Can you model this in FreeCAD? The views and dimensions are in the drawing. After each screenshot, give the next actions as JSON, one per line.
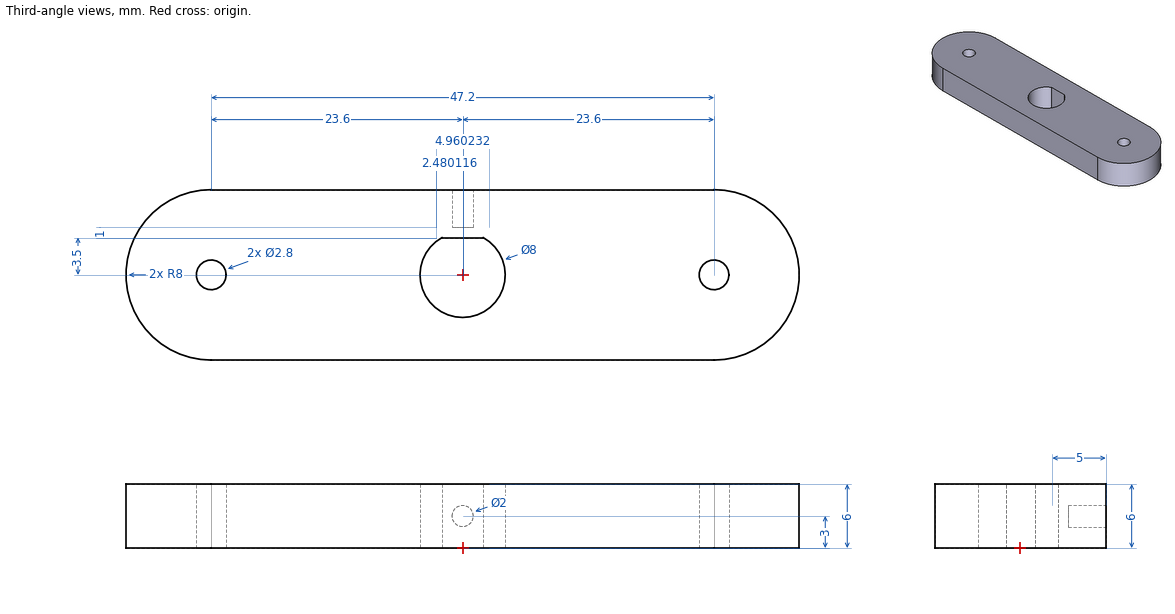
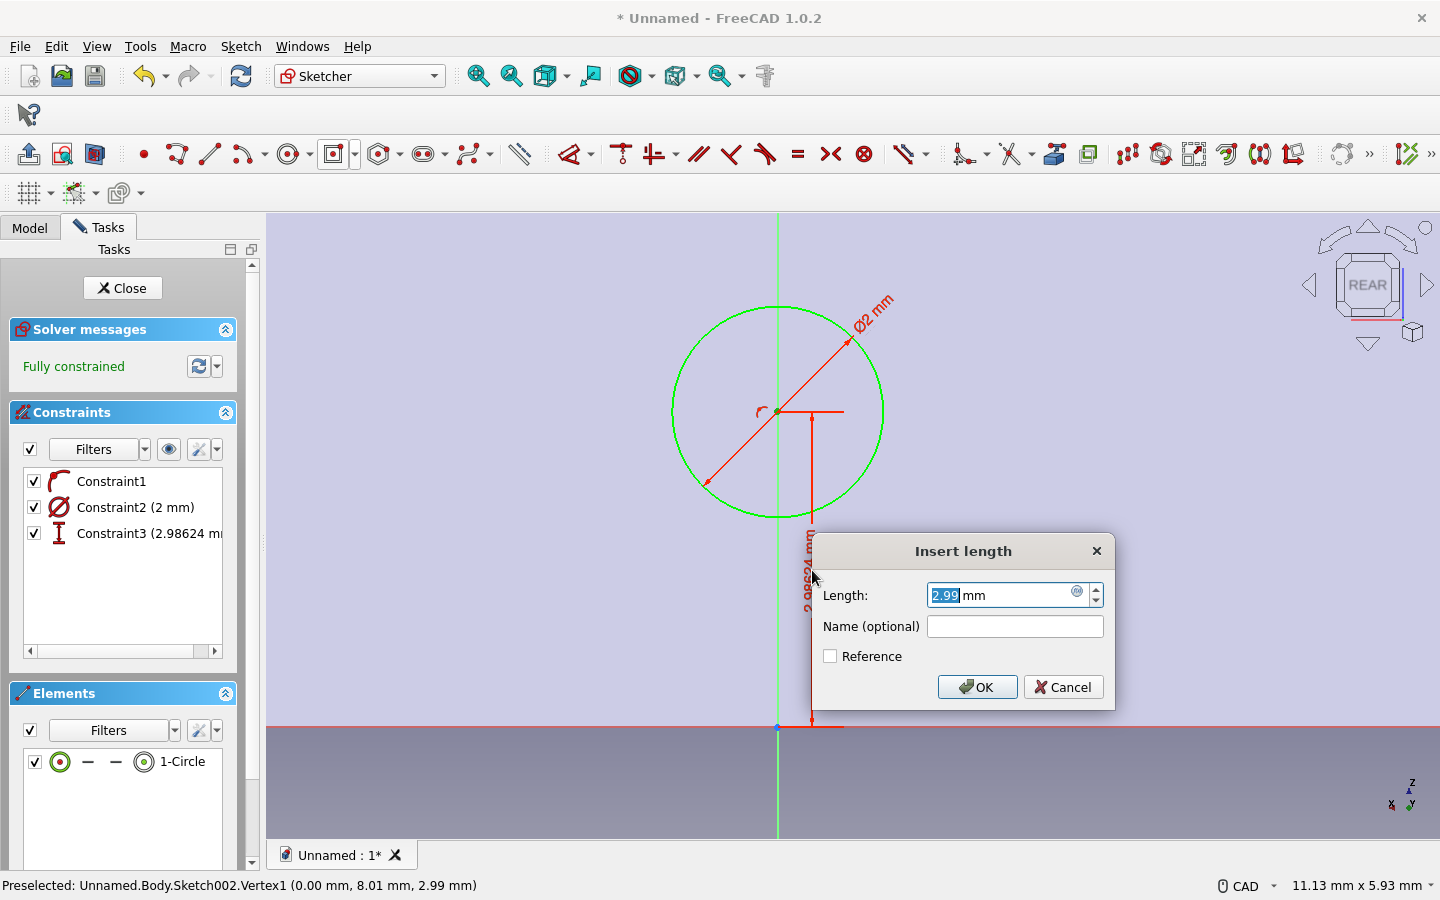
{"action": "type", "text": "3"}
{"action": "key", "text": "Return"}
{"action": "key", "text": "Escape"}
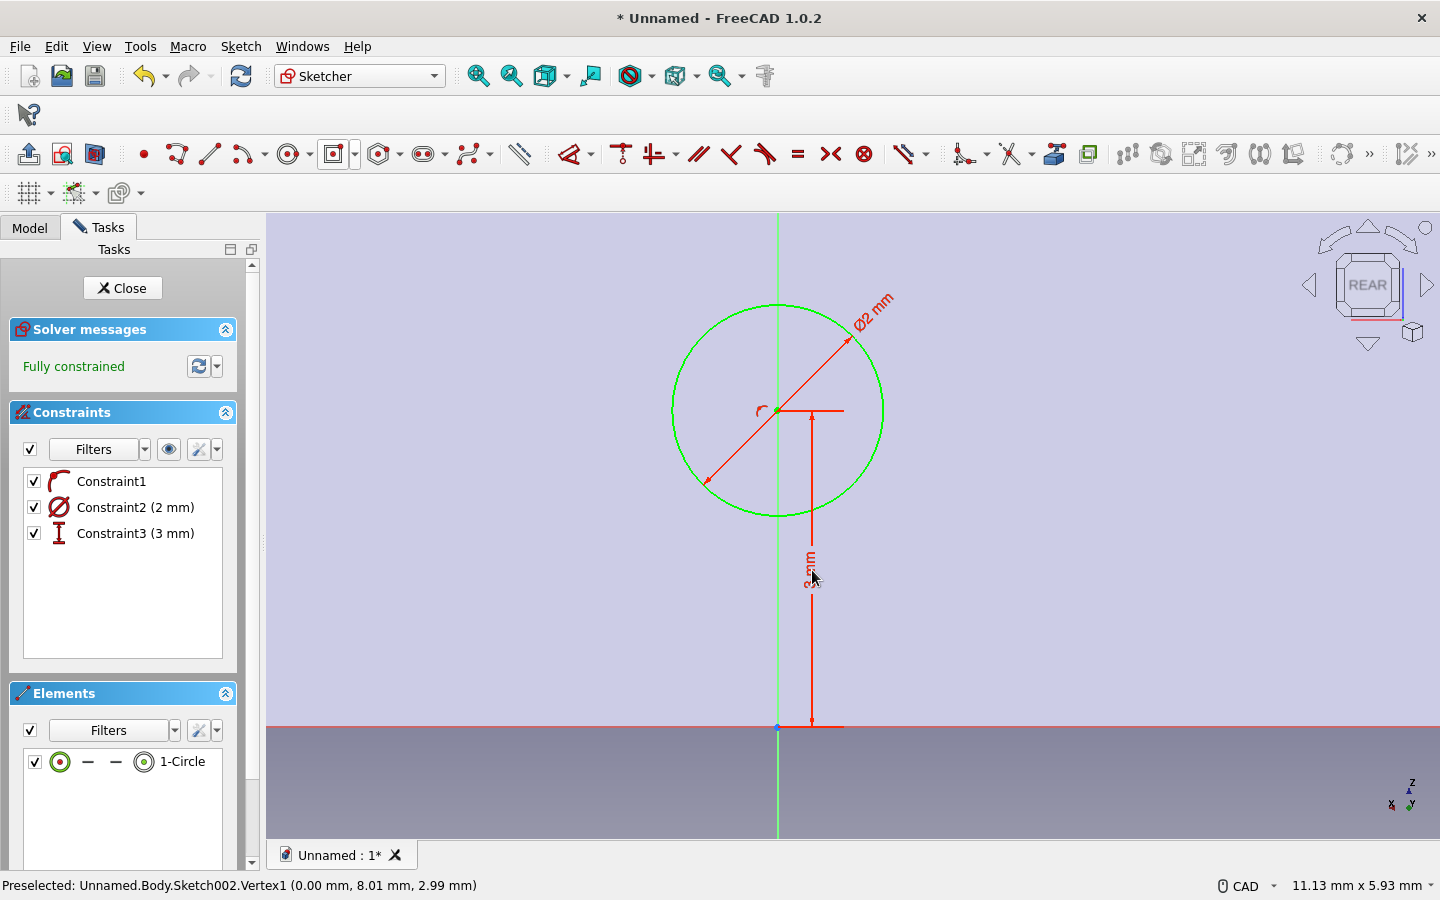
{"action": "left_click", "coordinate": [123, 288]}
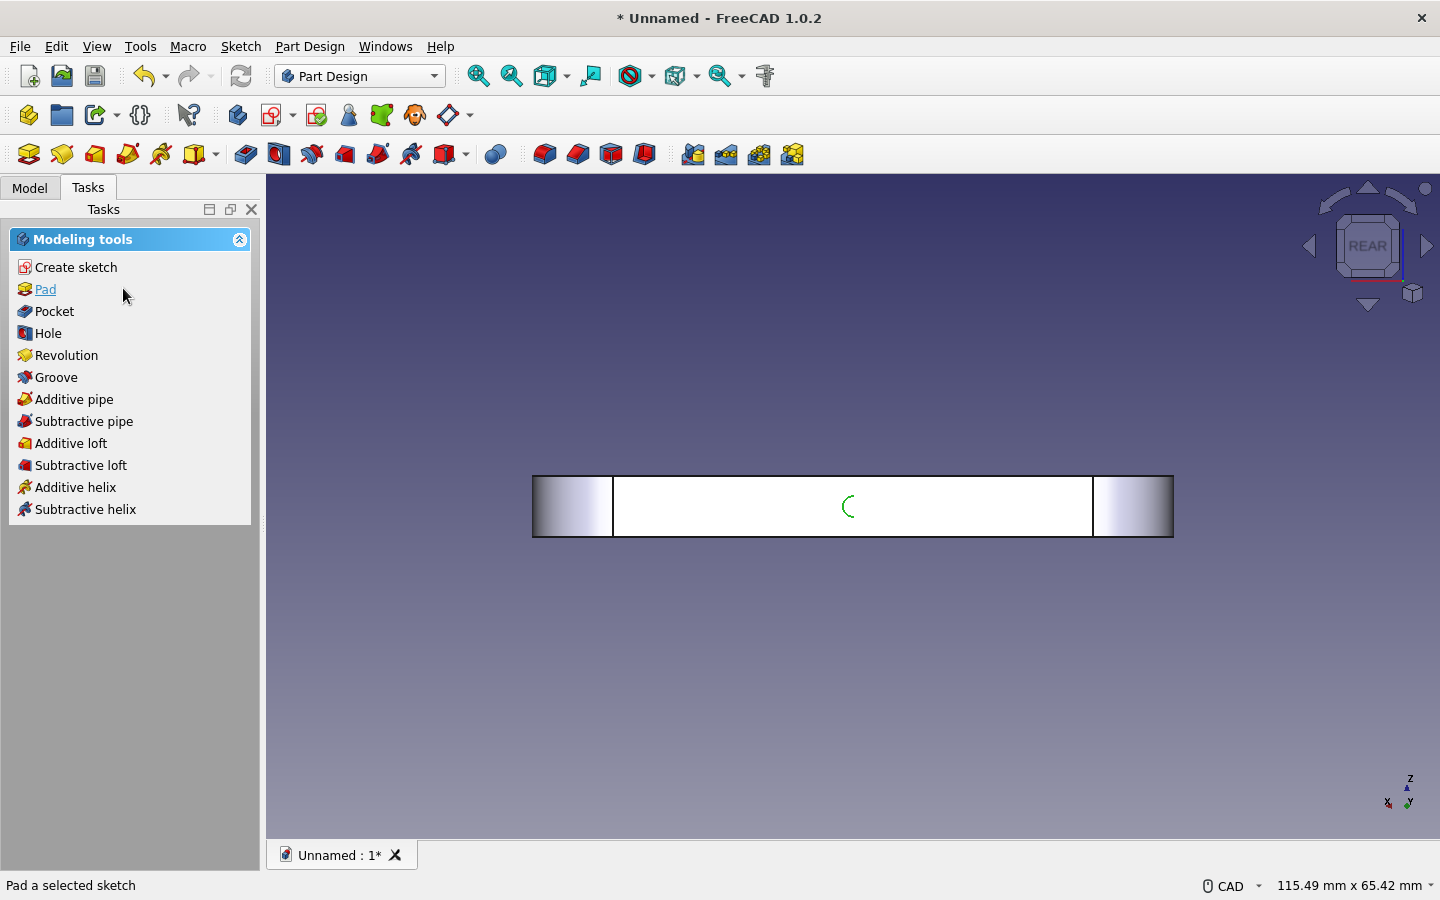
{"action": "left_click", "coordinate": [246, 154]}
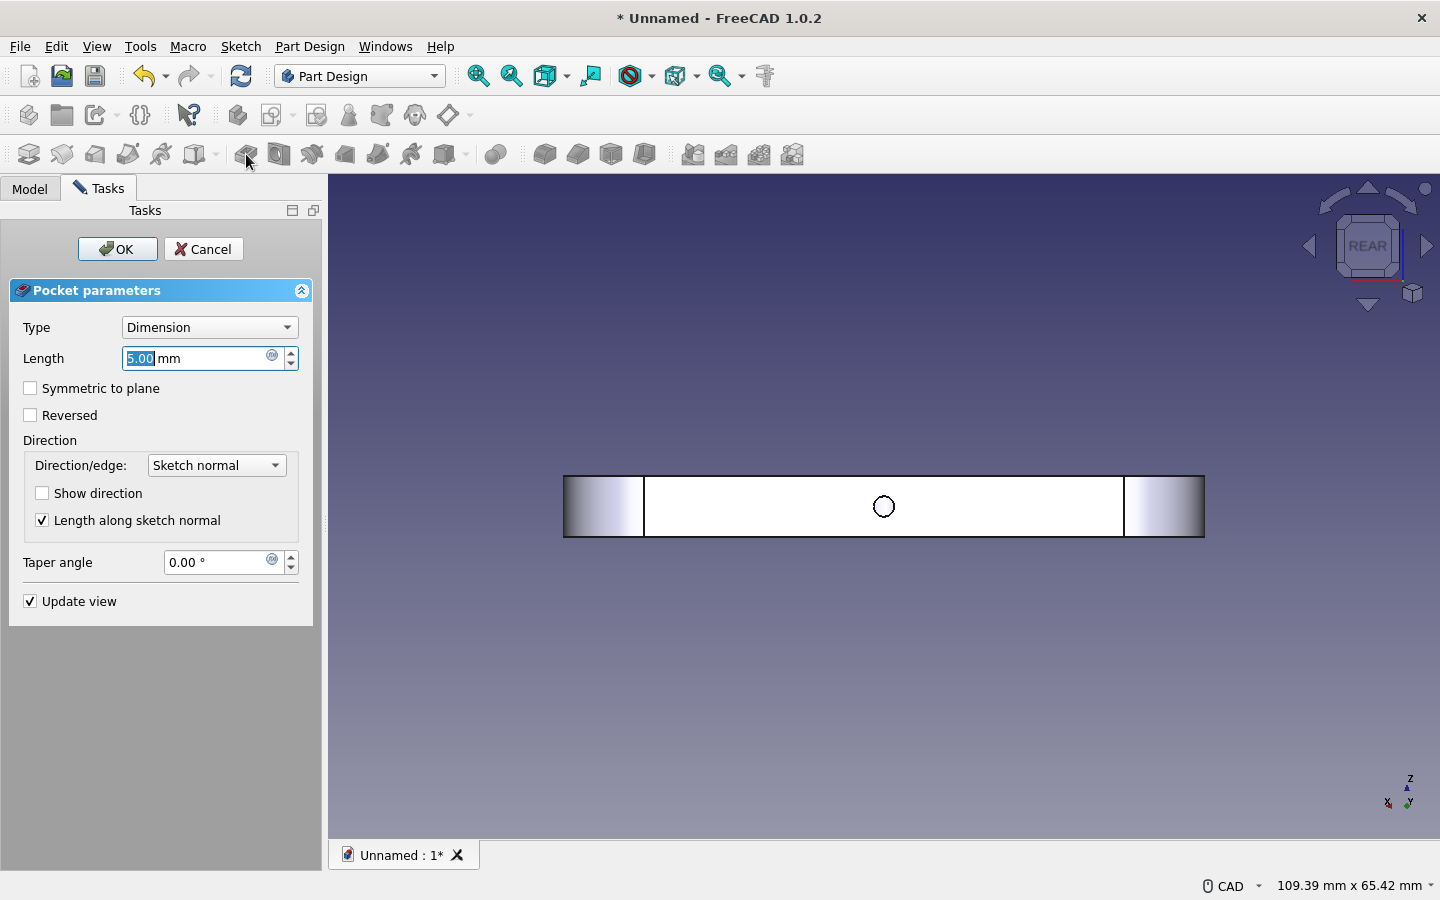
{"action": "type", "text": "5"}
{"action": "key", "text": "Tab"}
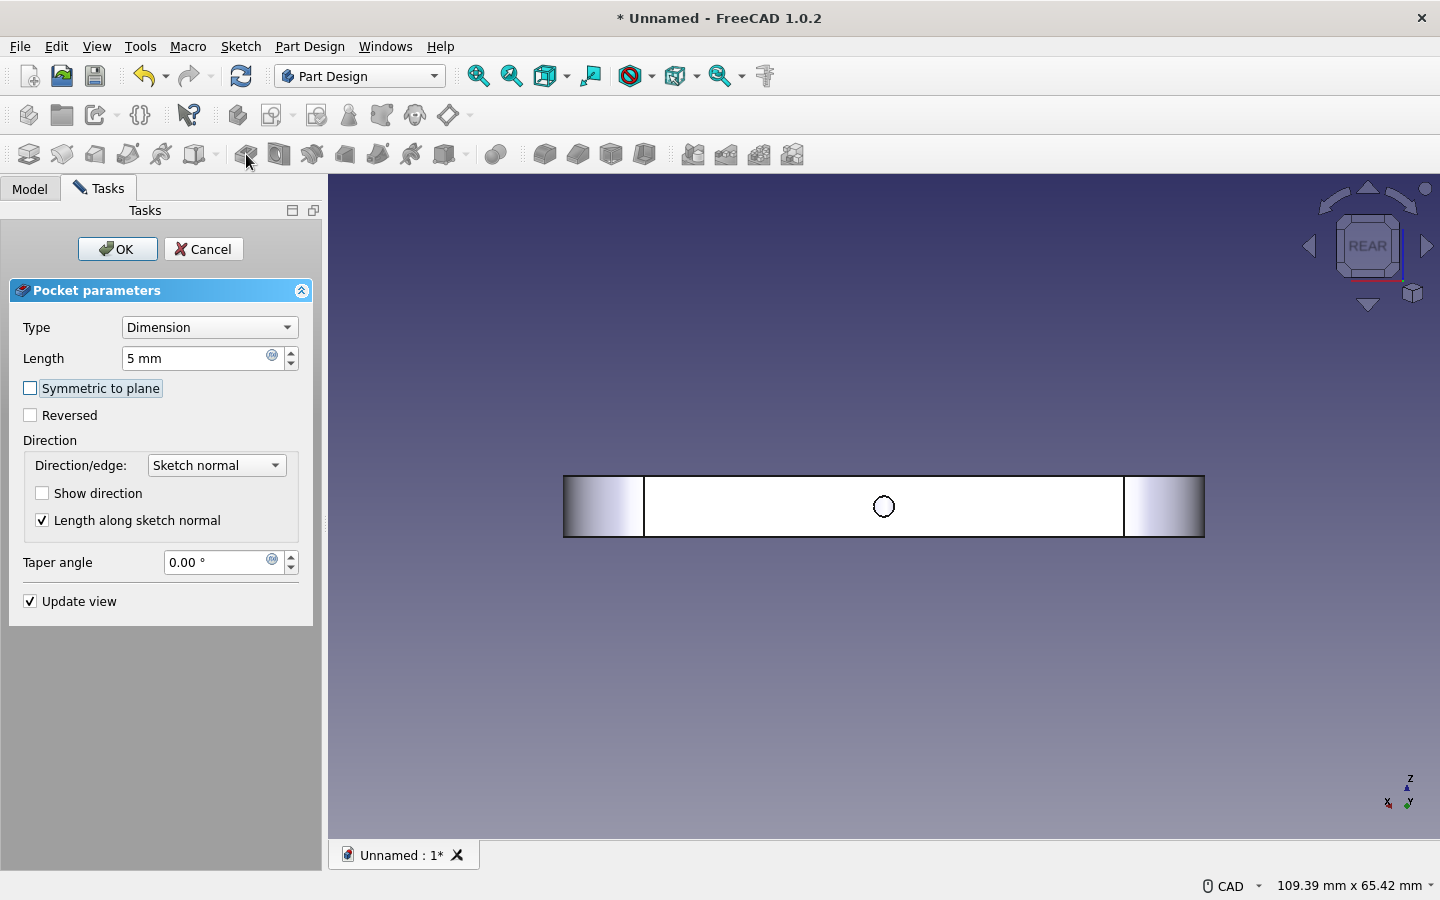
{"action": "left_click", "coordinate": [118, 249]}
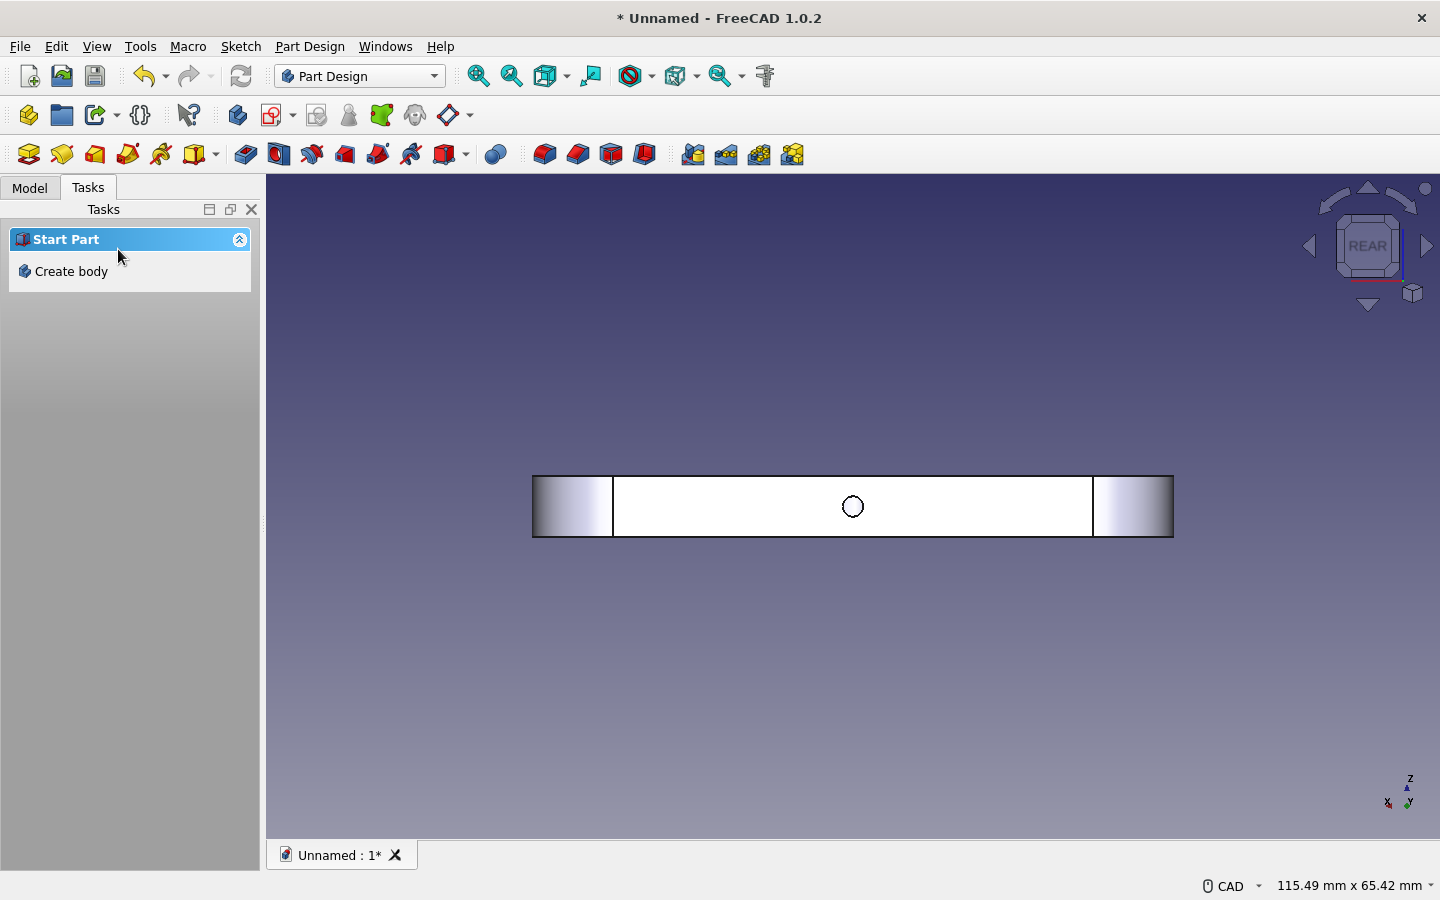
{"action": "key", "text": "5"}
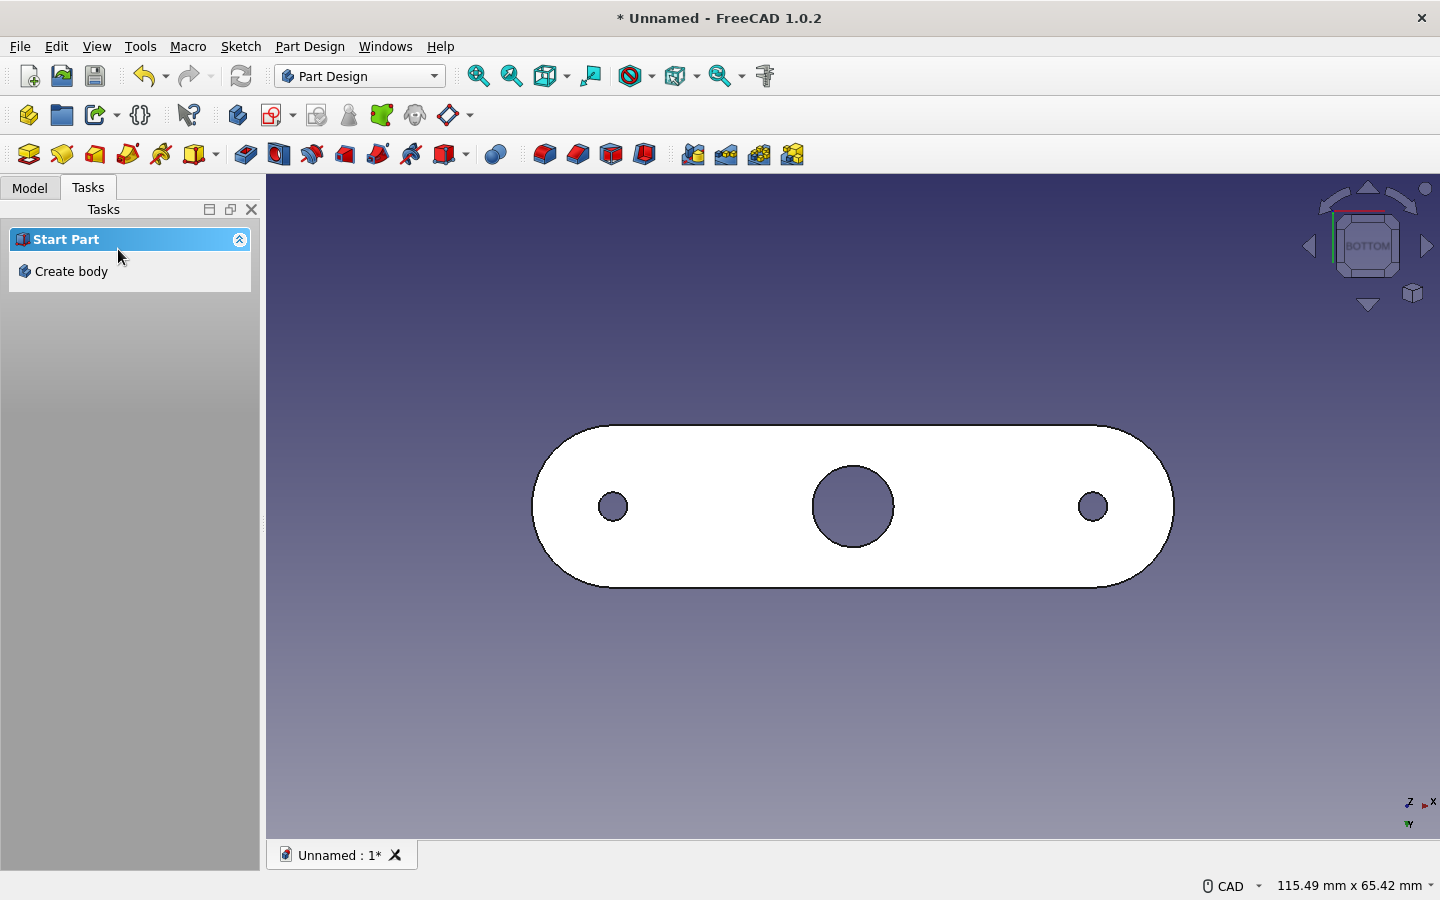
{"action": "left_click", "coordinate": [945, 482]}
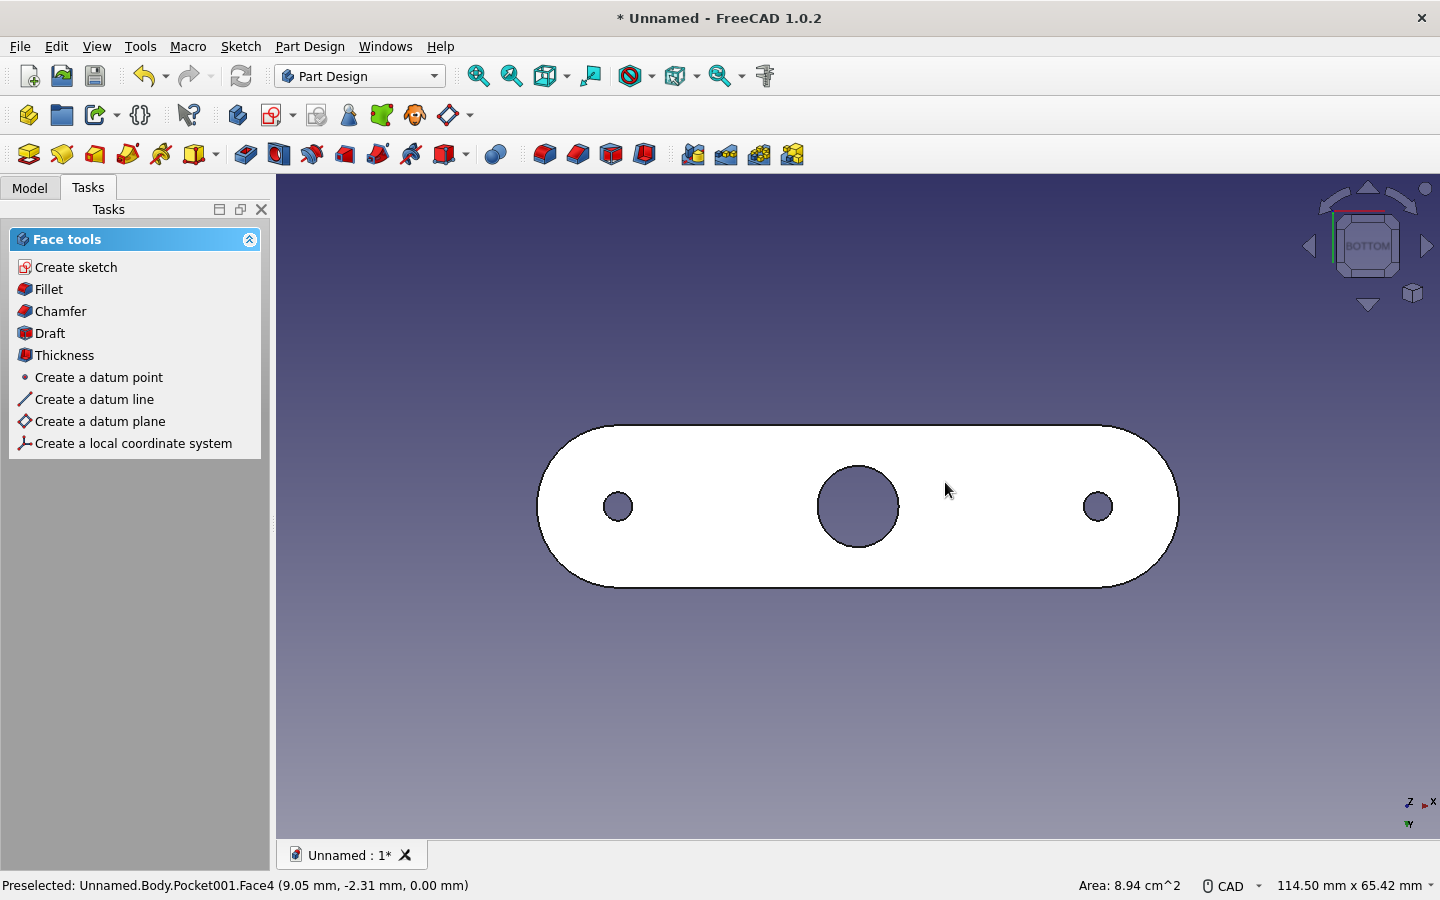
{"action": "left_click", "coordinate": [270, 116]}